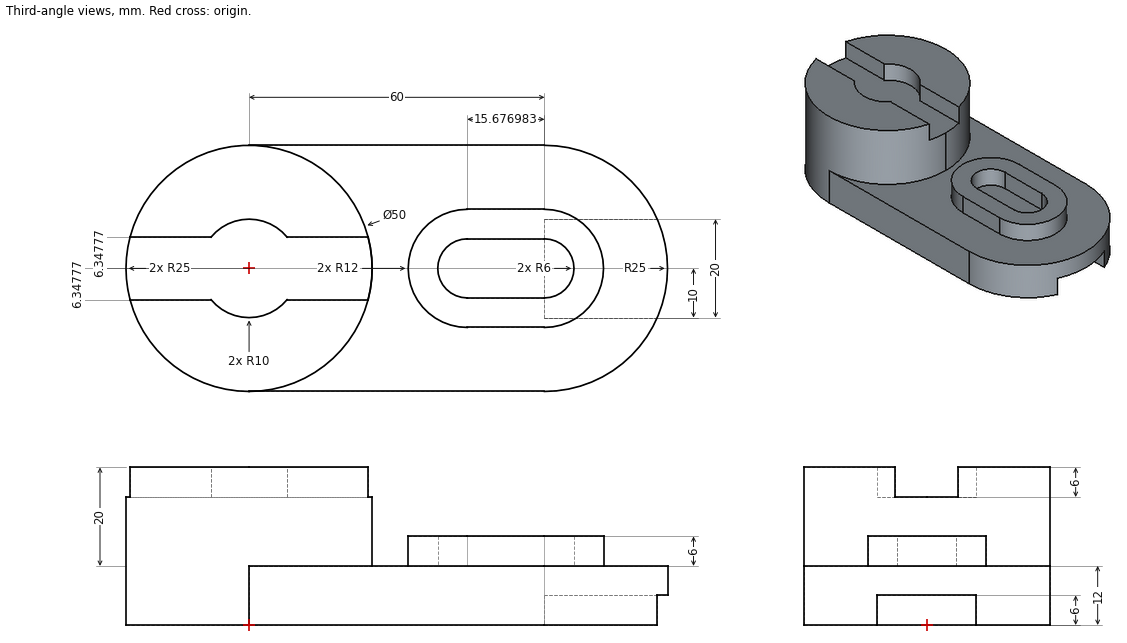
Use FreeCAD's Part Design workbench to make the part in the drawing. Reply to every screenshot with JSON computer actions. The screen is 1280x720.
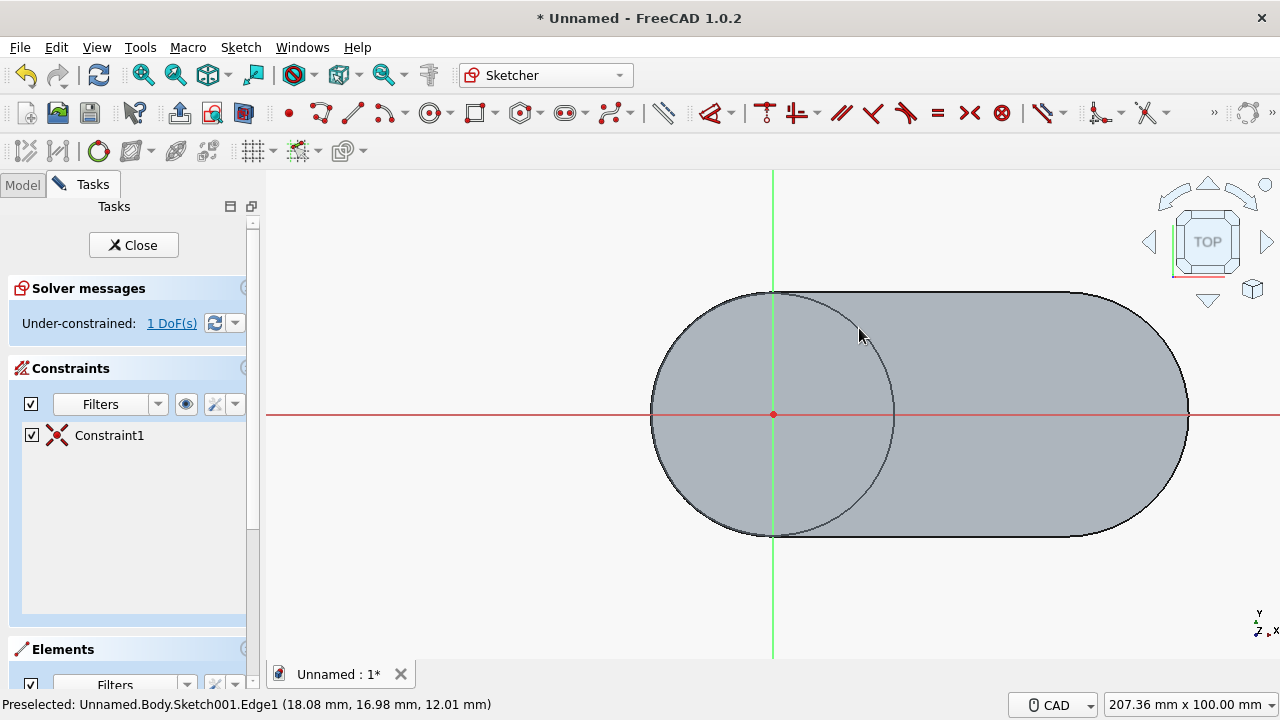
{"action": "key", "text": "d"}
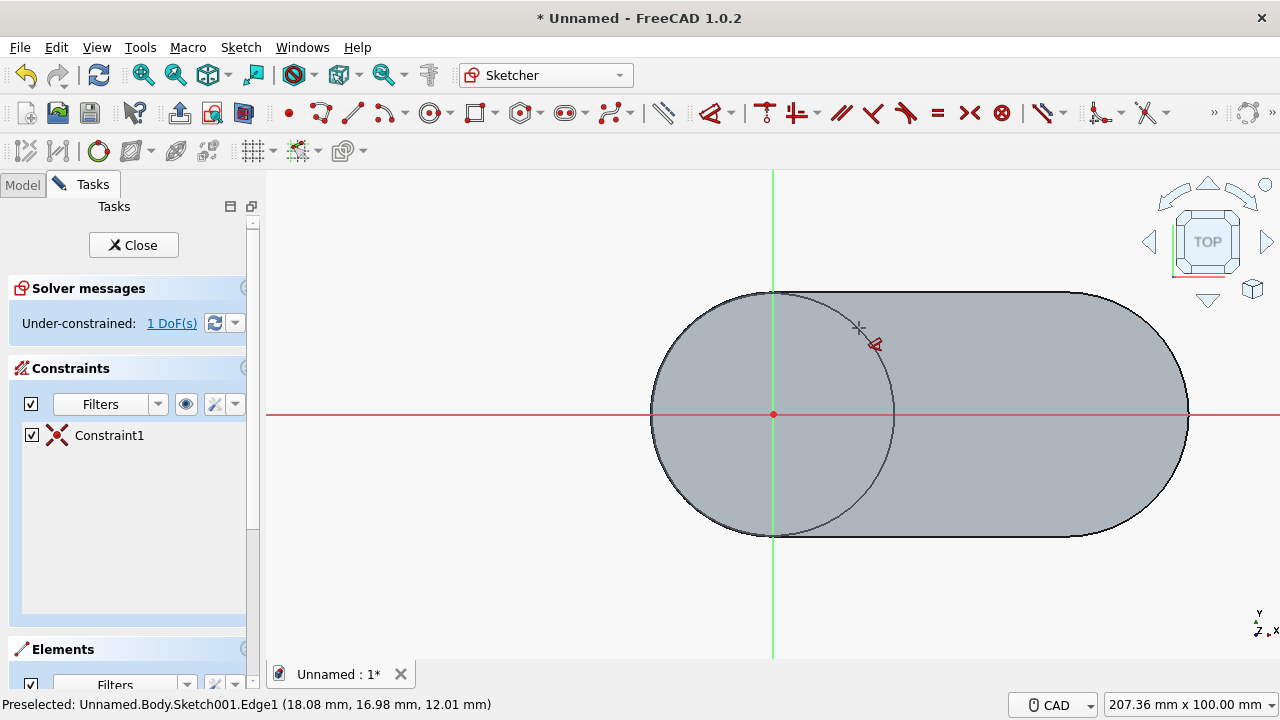
{"action": "left_click", "coordinate": [858, 328]}
{"action": "left_click", "coordinate": [880, 305]}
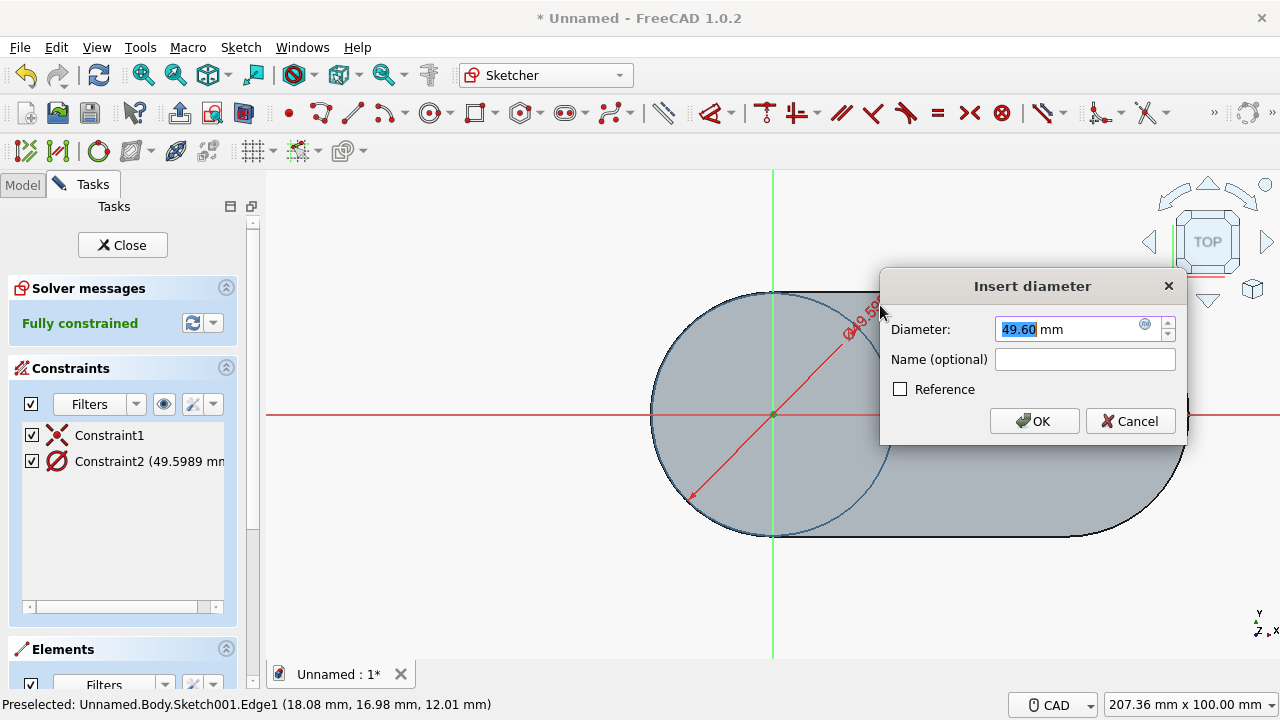
{"action": "type", "text": "50"}
{"action": "key", "text": "Return"}
{"action": "key", "text": "Escape"}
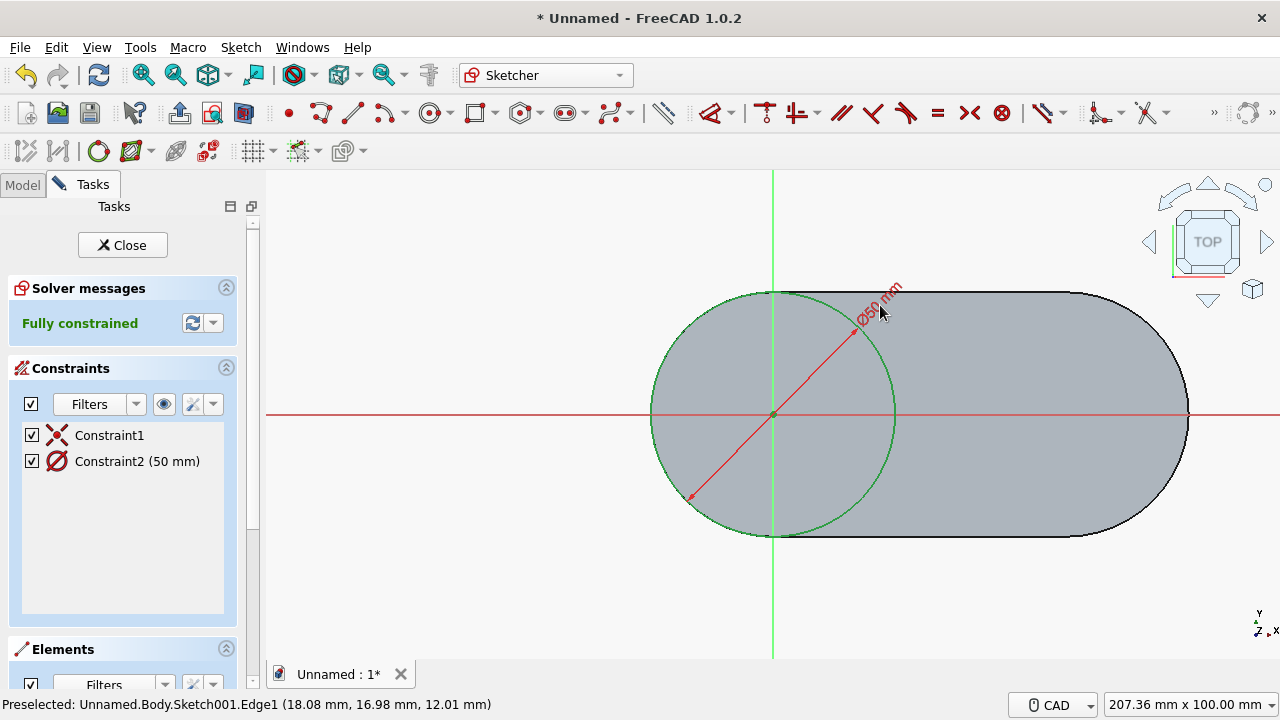
{"action": "left_click", "coordinate": [123, 245]}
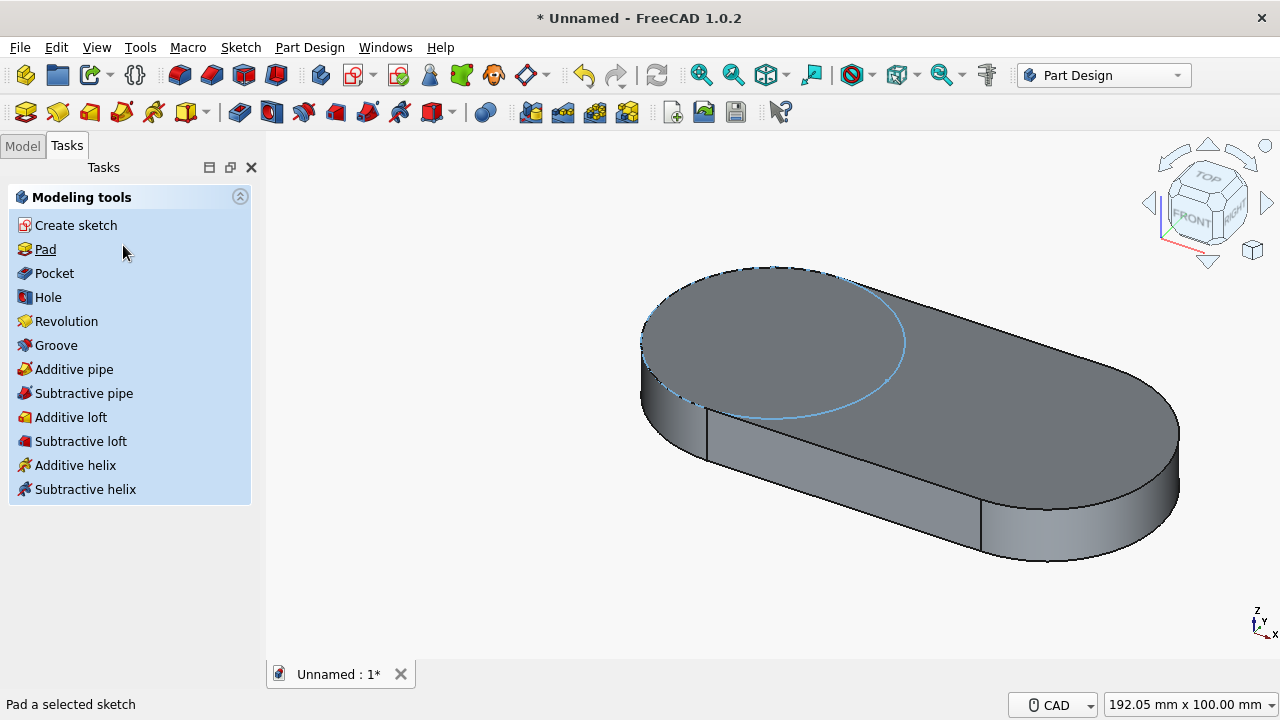
{"action": "left_click", "coordinate": [26, 112]}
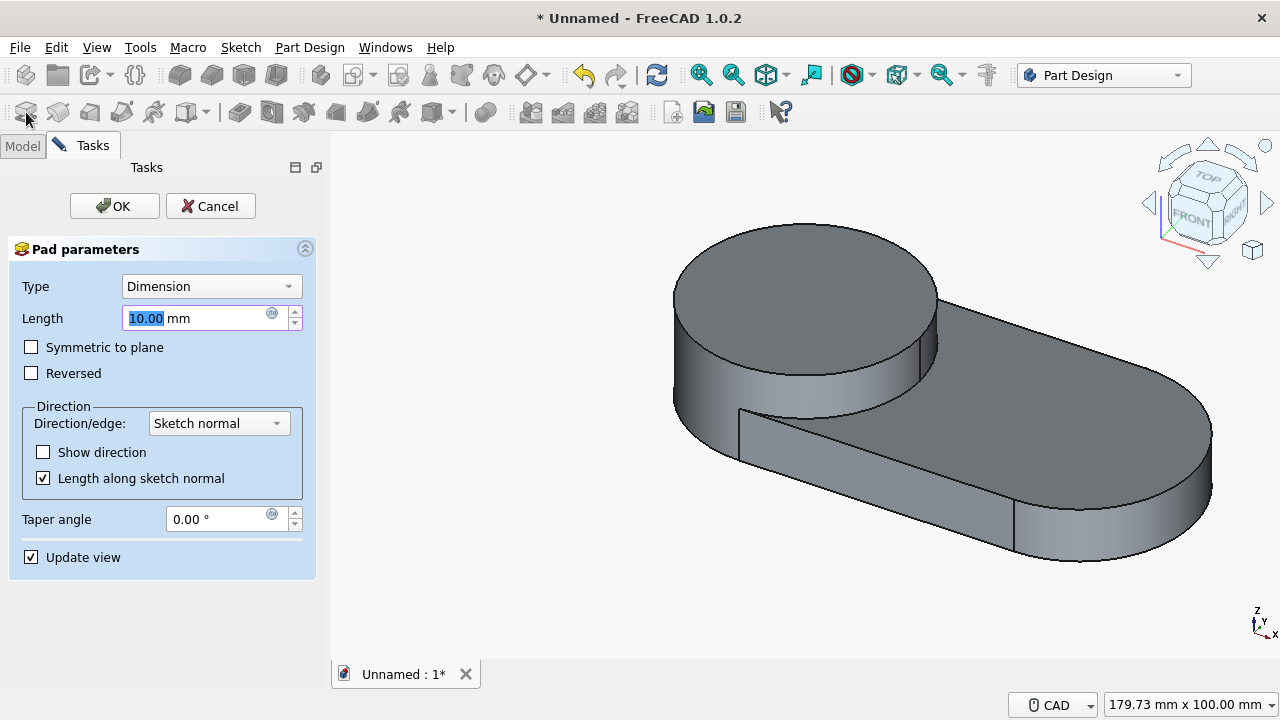
{"action": "type", "text": "20"}
{"action": "key", "text": "Tab"}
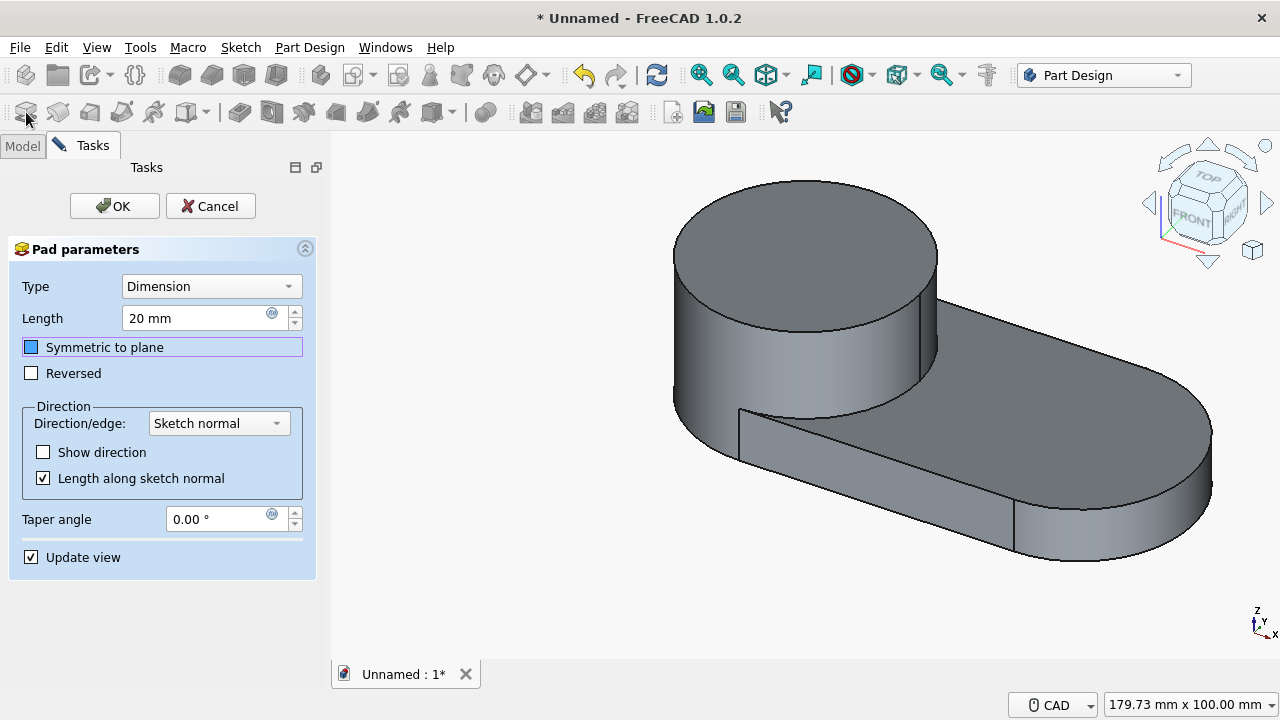
{"action": "left_click", "coordinate": [115, 206]}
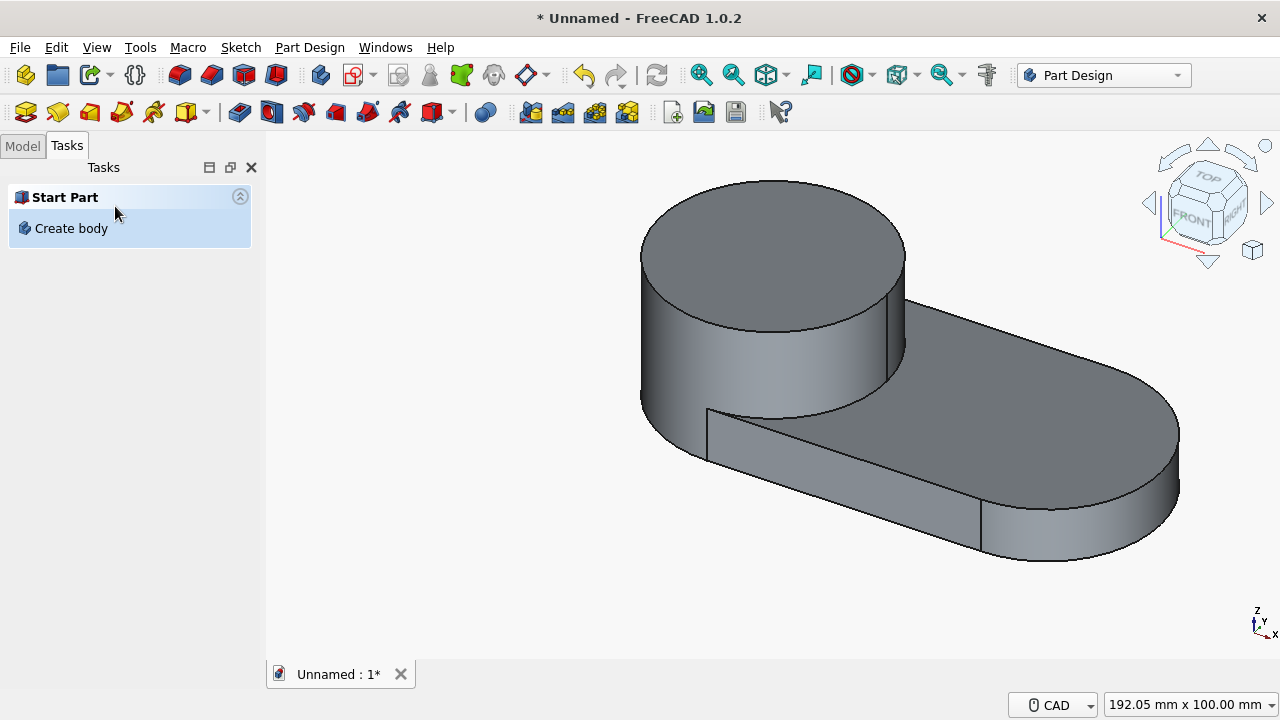
{"action": "left_click", "coordinate": [23, 145]}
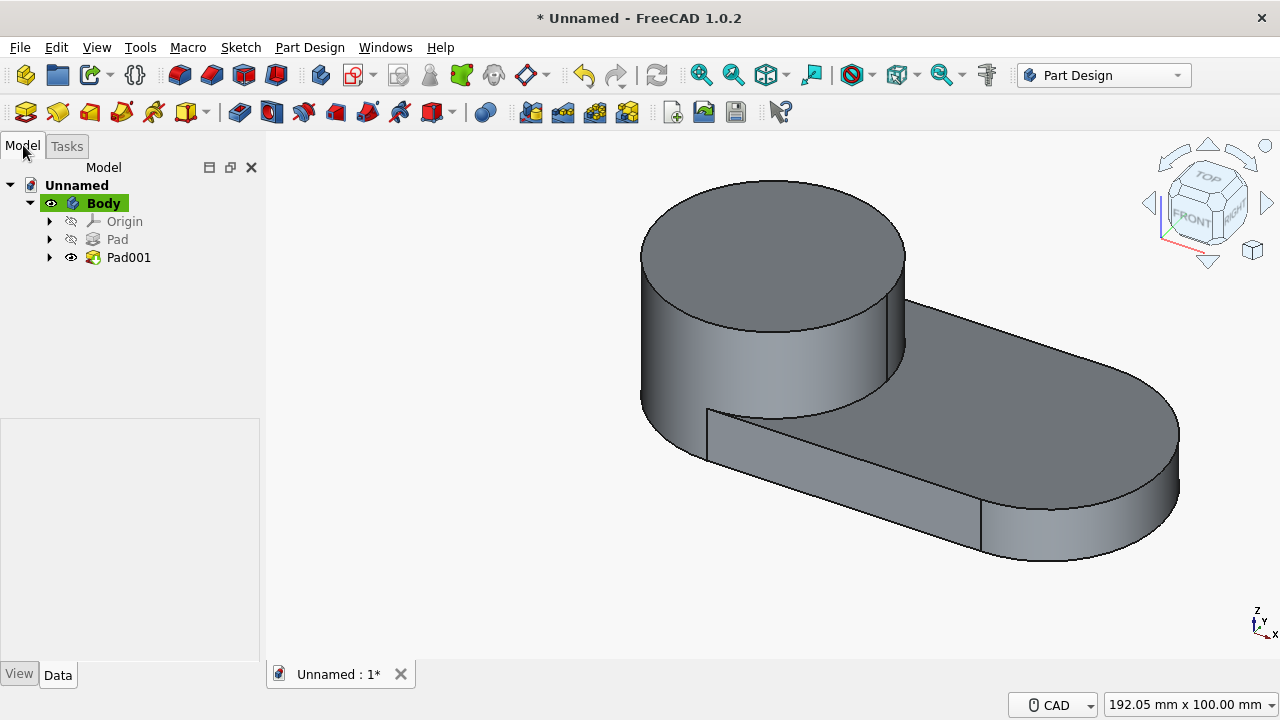
{"action": "left_click", "coordinate": [50, 221]}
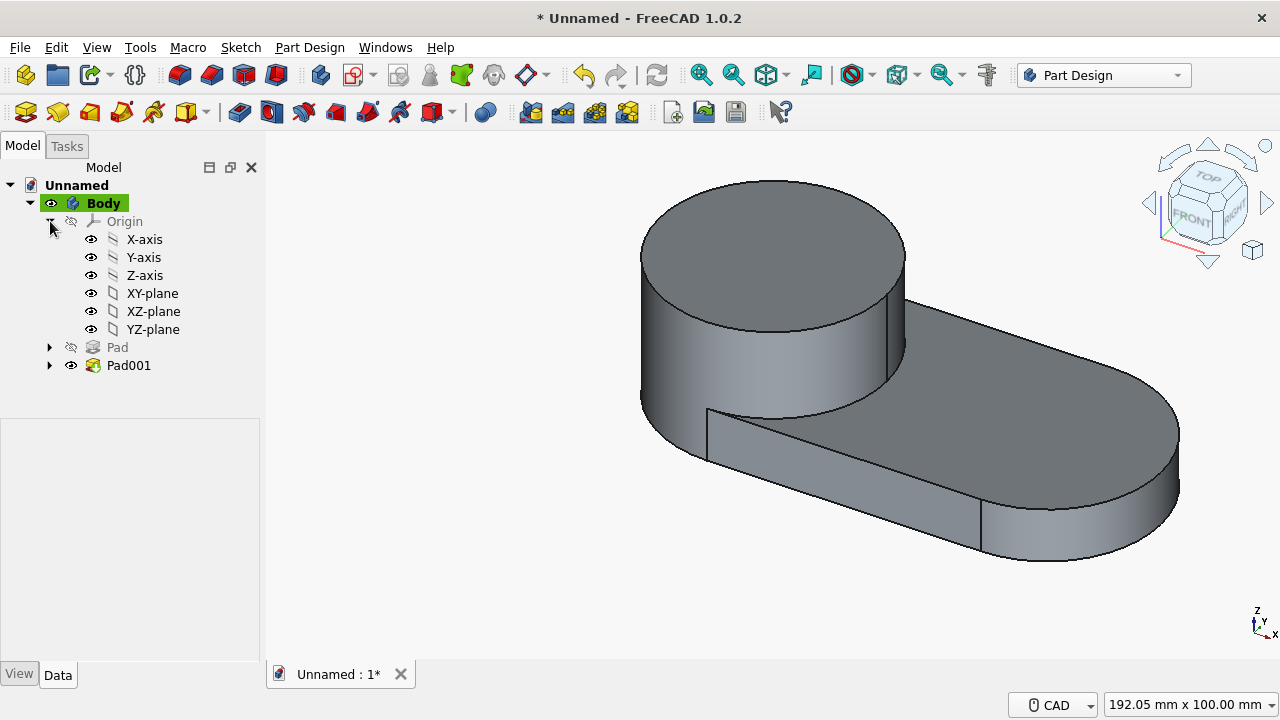
{"action": "left_click", "coordinate": [136, 293]}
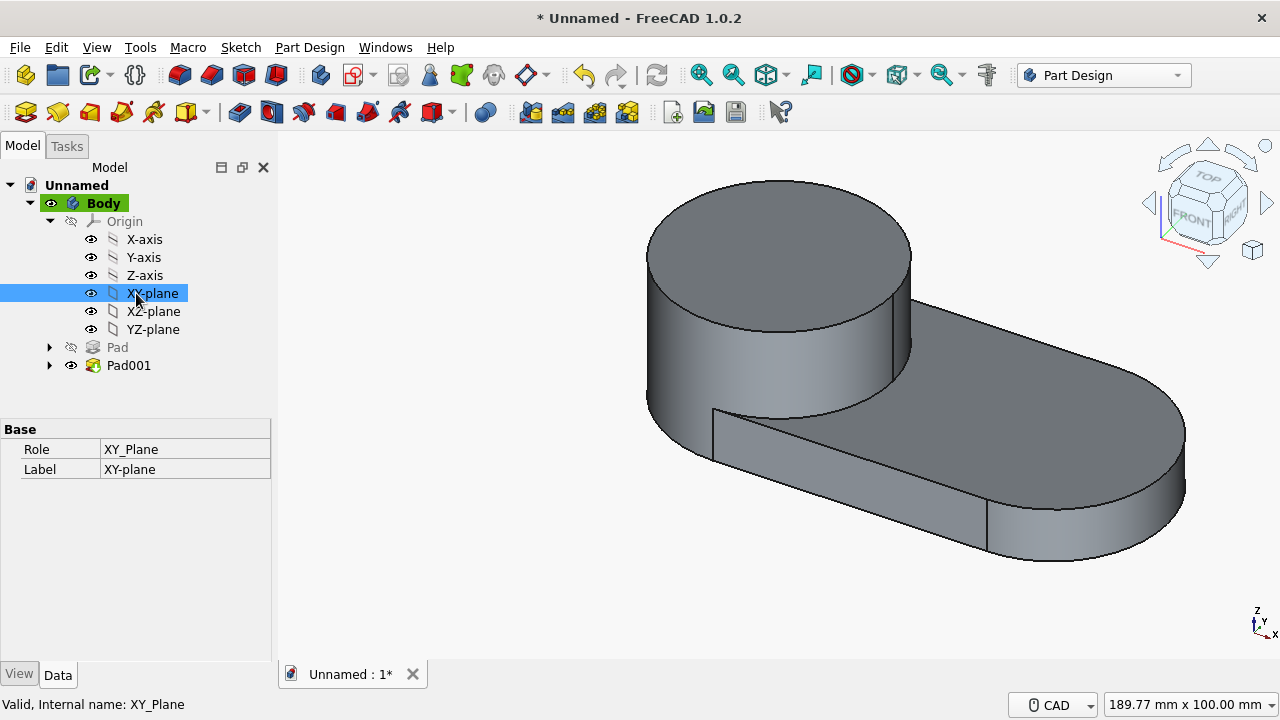
{"action": "left_click", "coordinate": [526, 76]}